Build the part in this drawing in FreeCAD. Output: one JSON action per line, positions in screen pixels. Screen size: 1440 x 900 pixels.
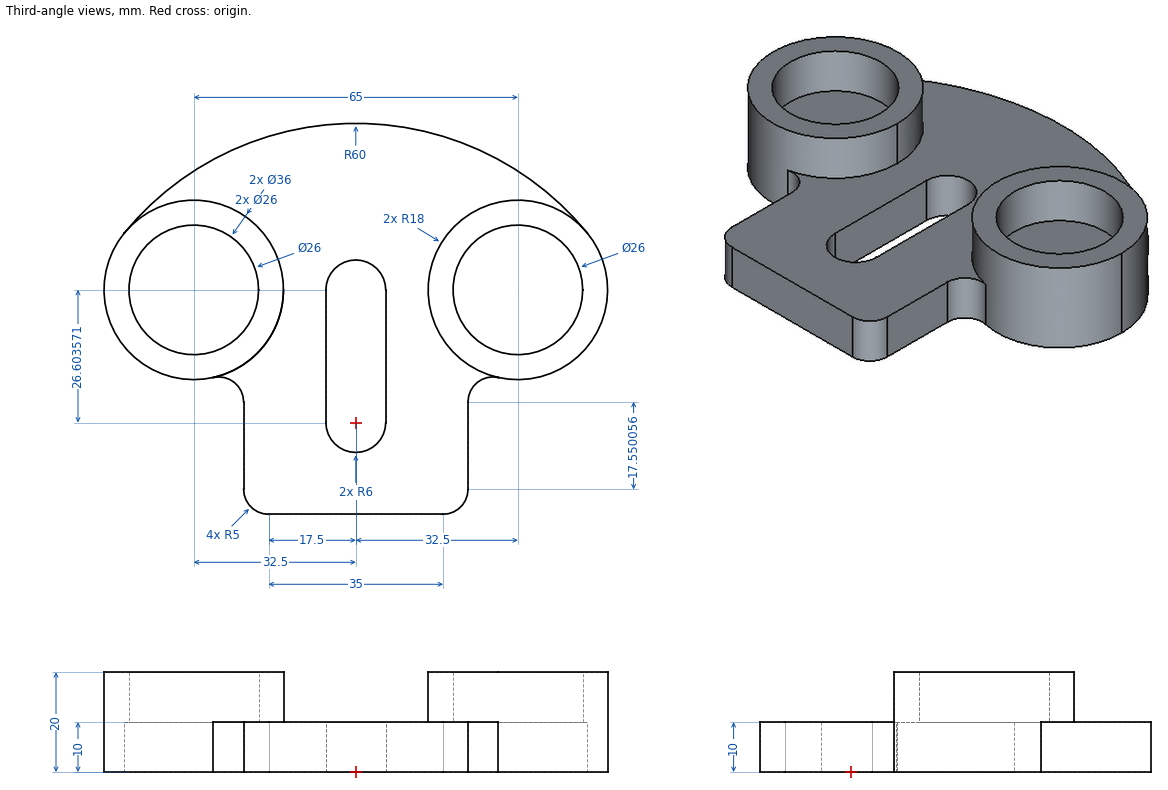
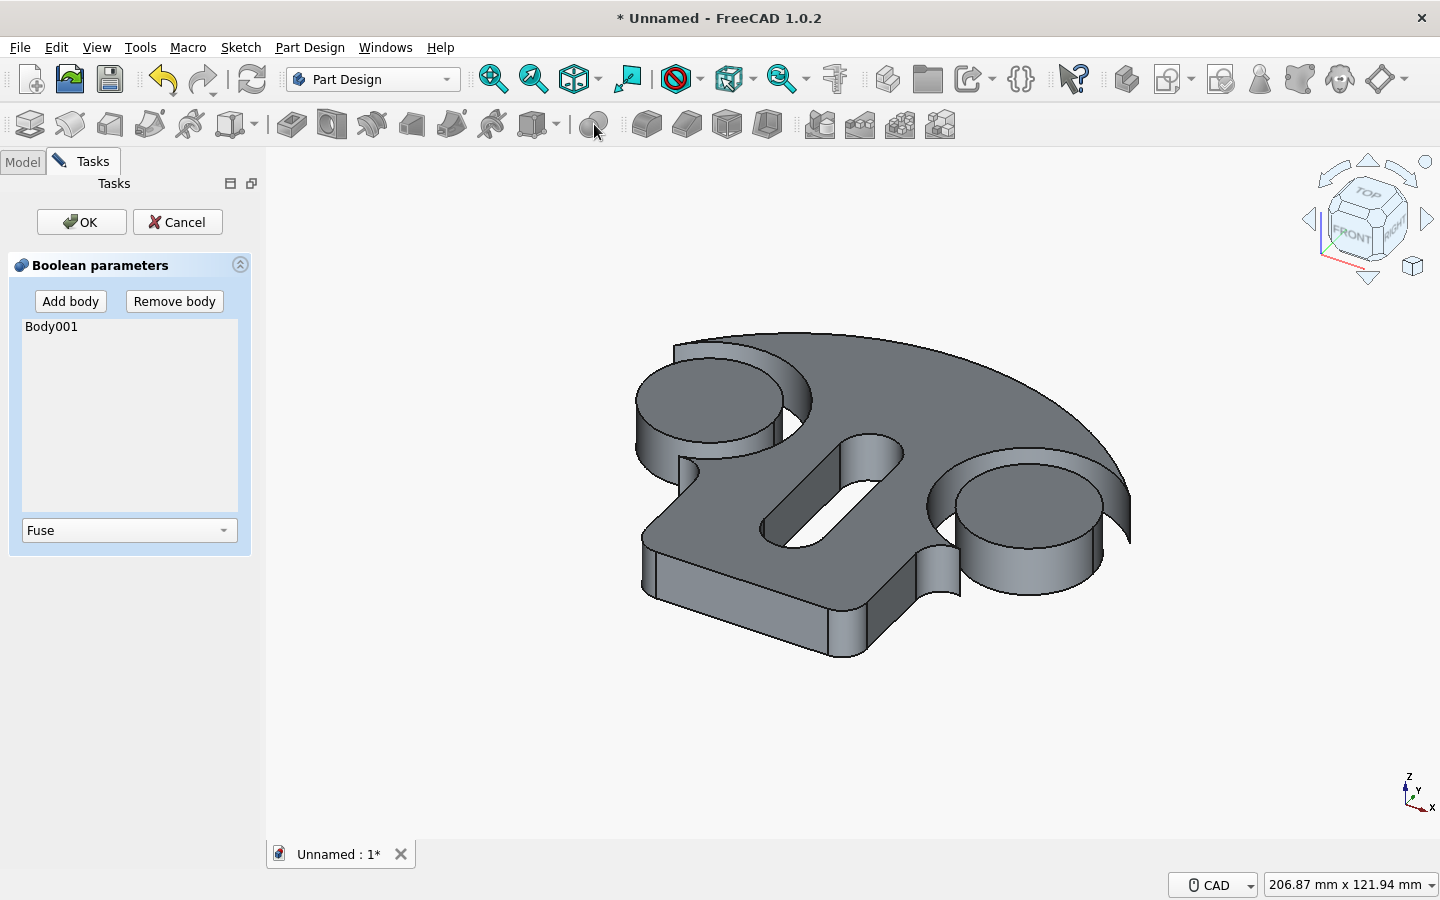
{"action": "left_click", "coordinate": [82, 222]}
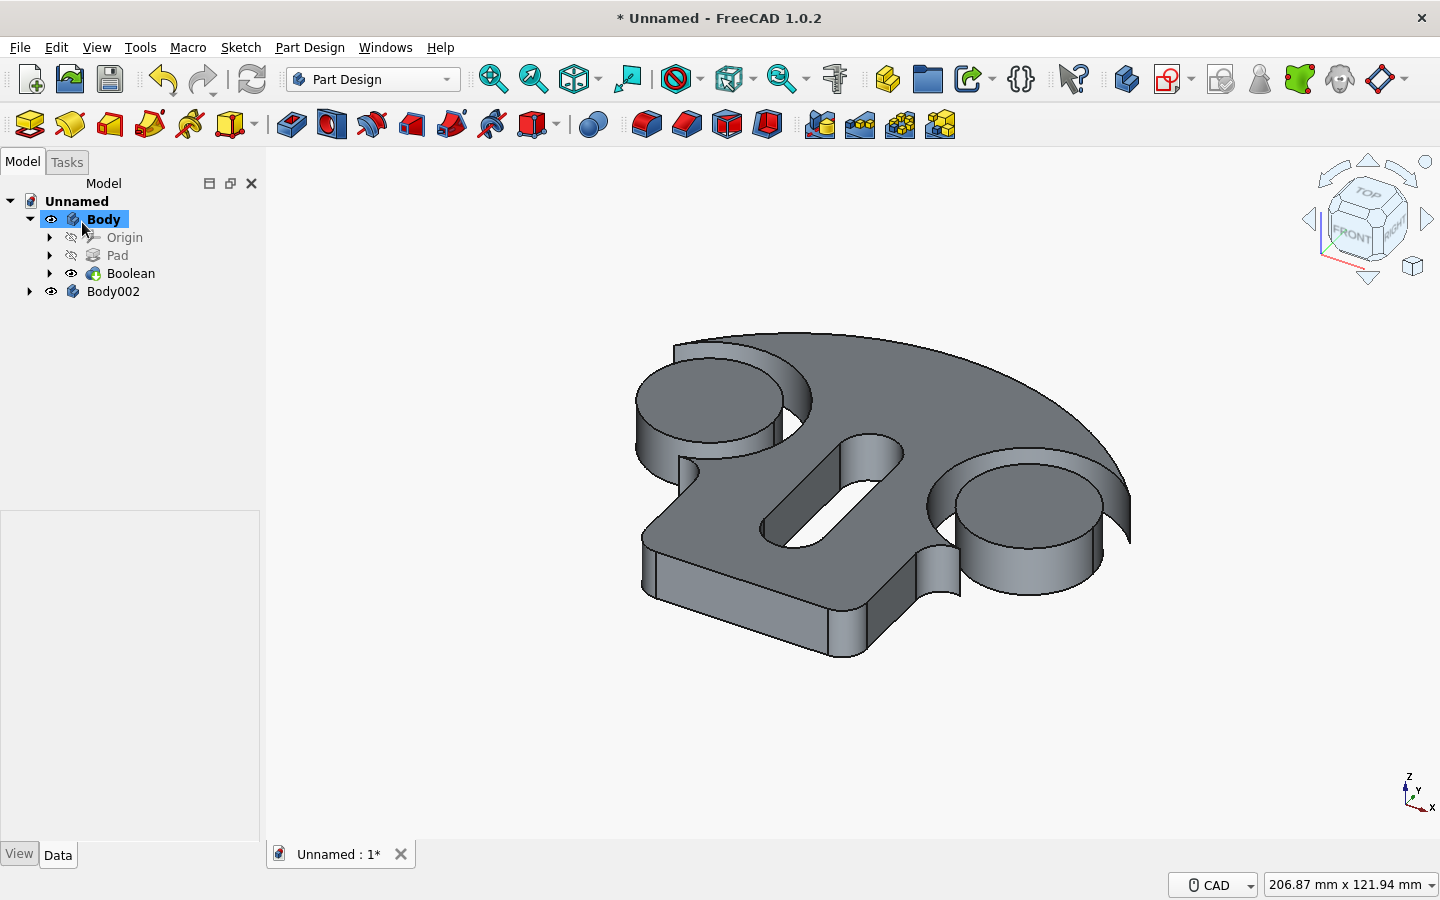
{"action": "left_click", "coordinate": [96, 291]}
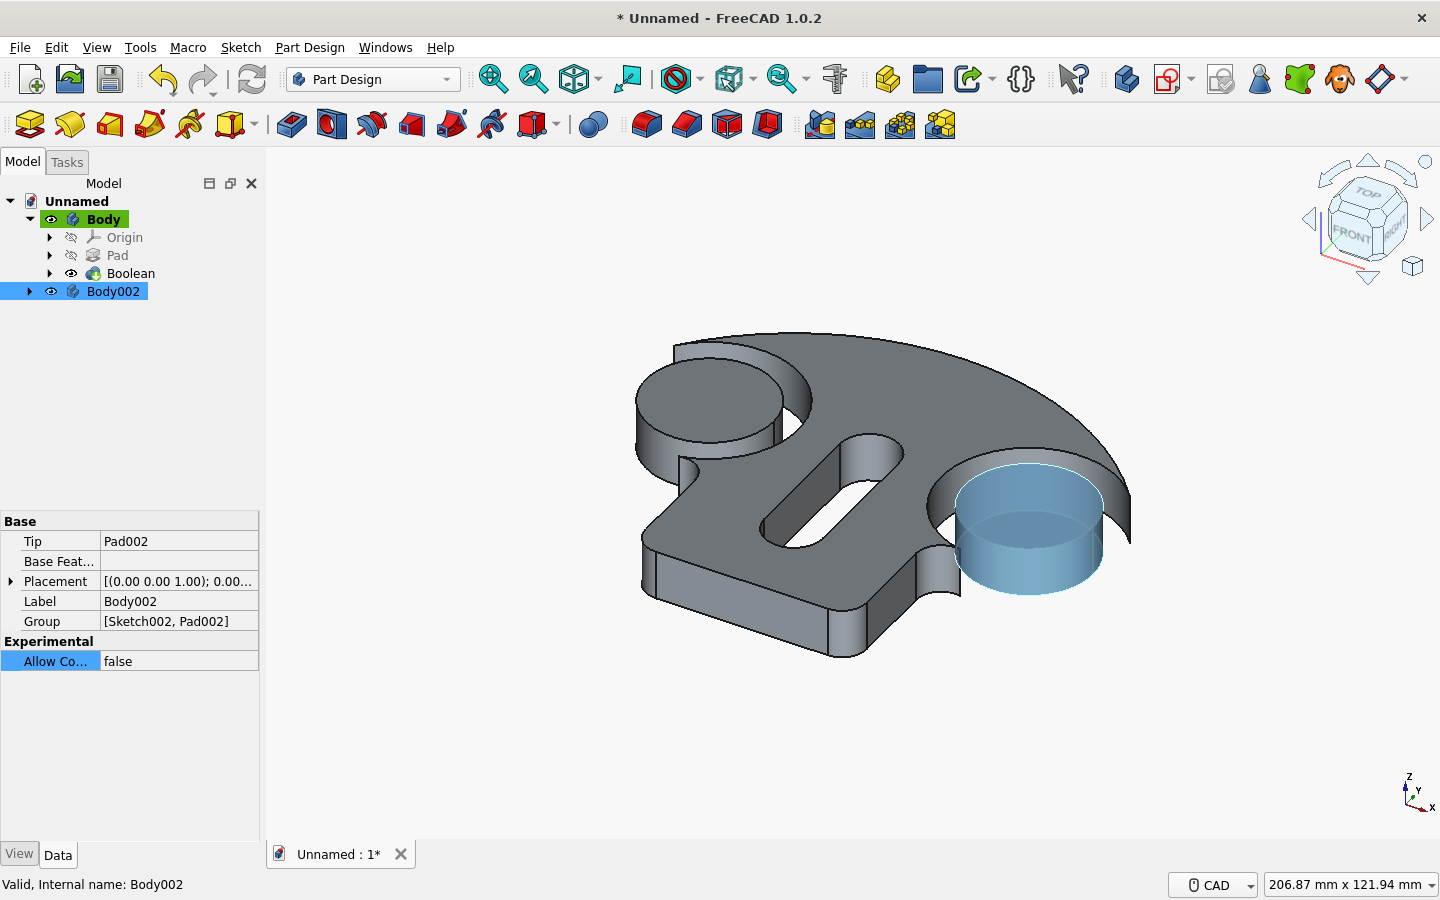
{"action": "left_click", "coordinate": [594, 124]}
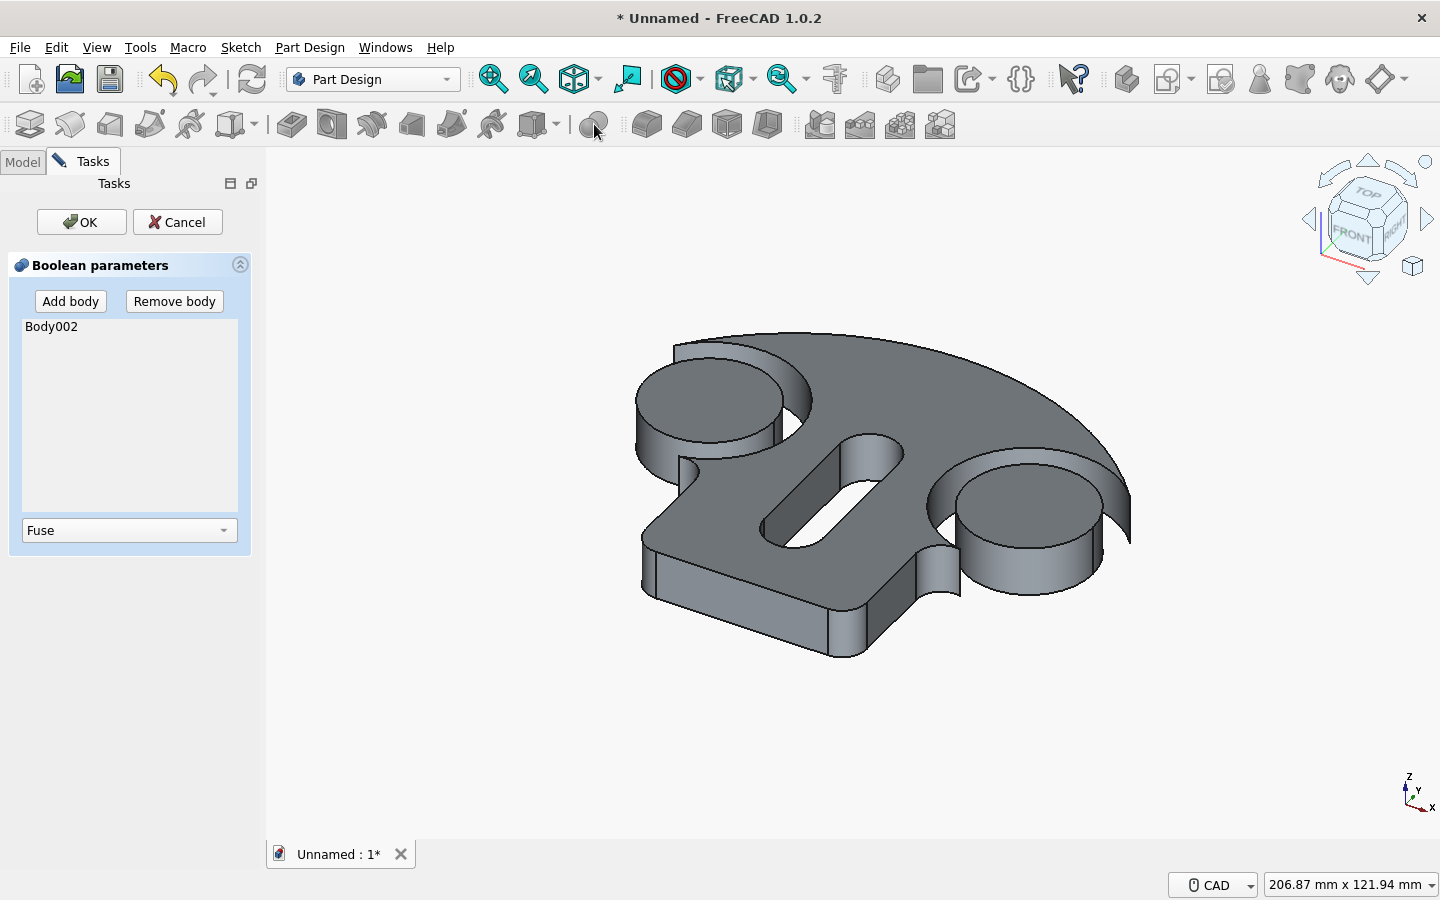
{"action": "left_click", "coordinate": [82, 222]}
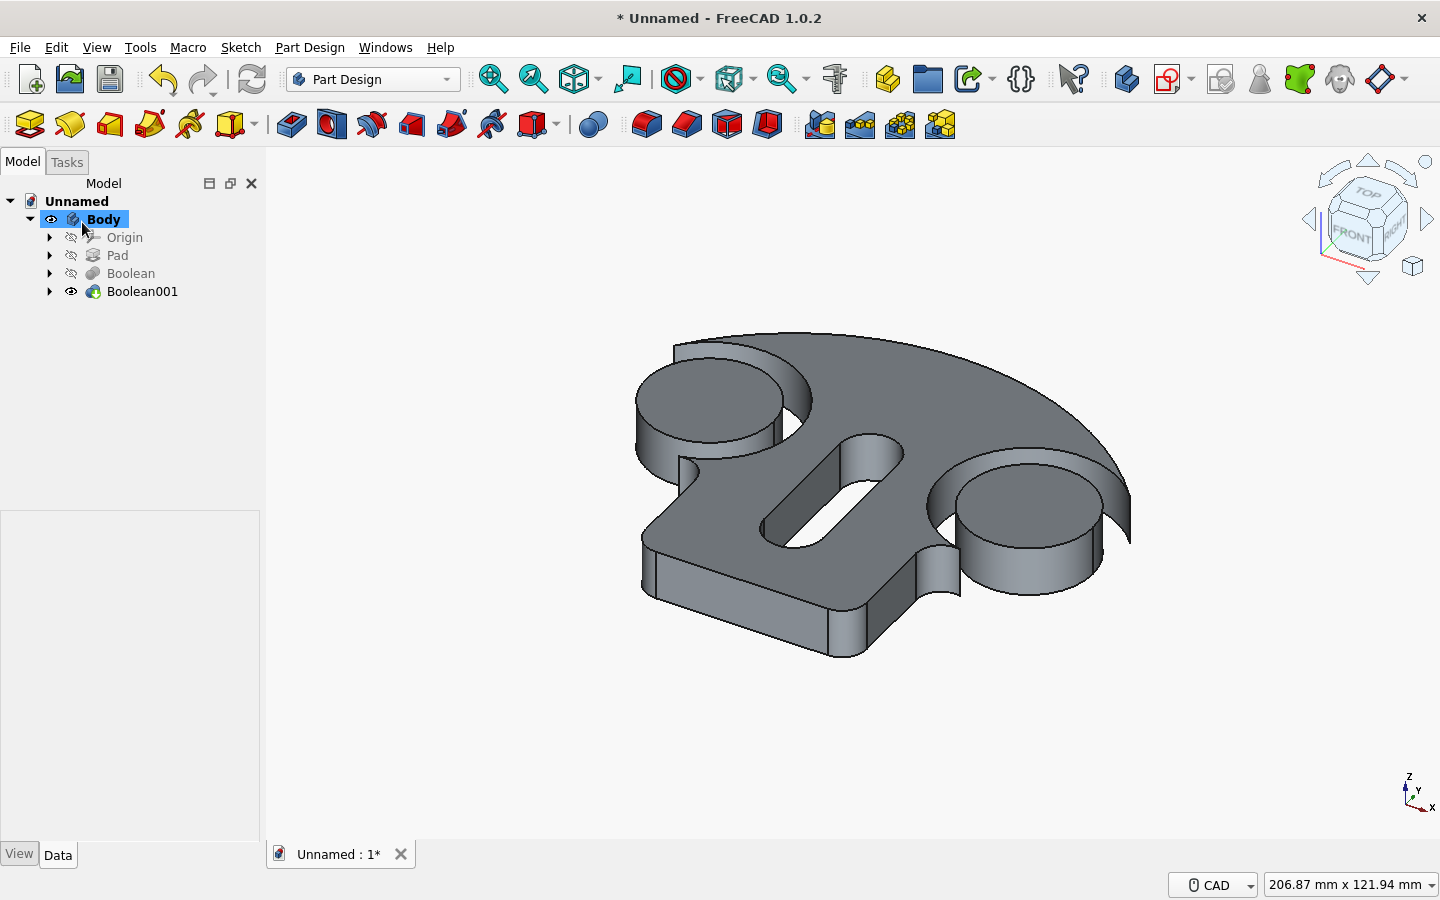
{"action": "left_click", "coordinate": [1168, 80]}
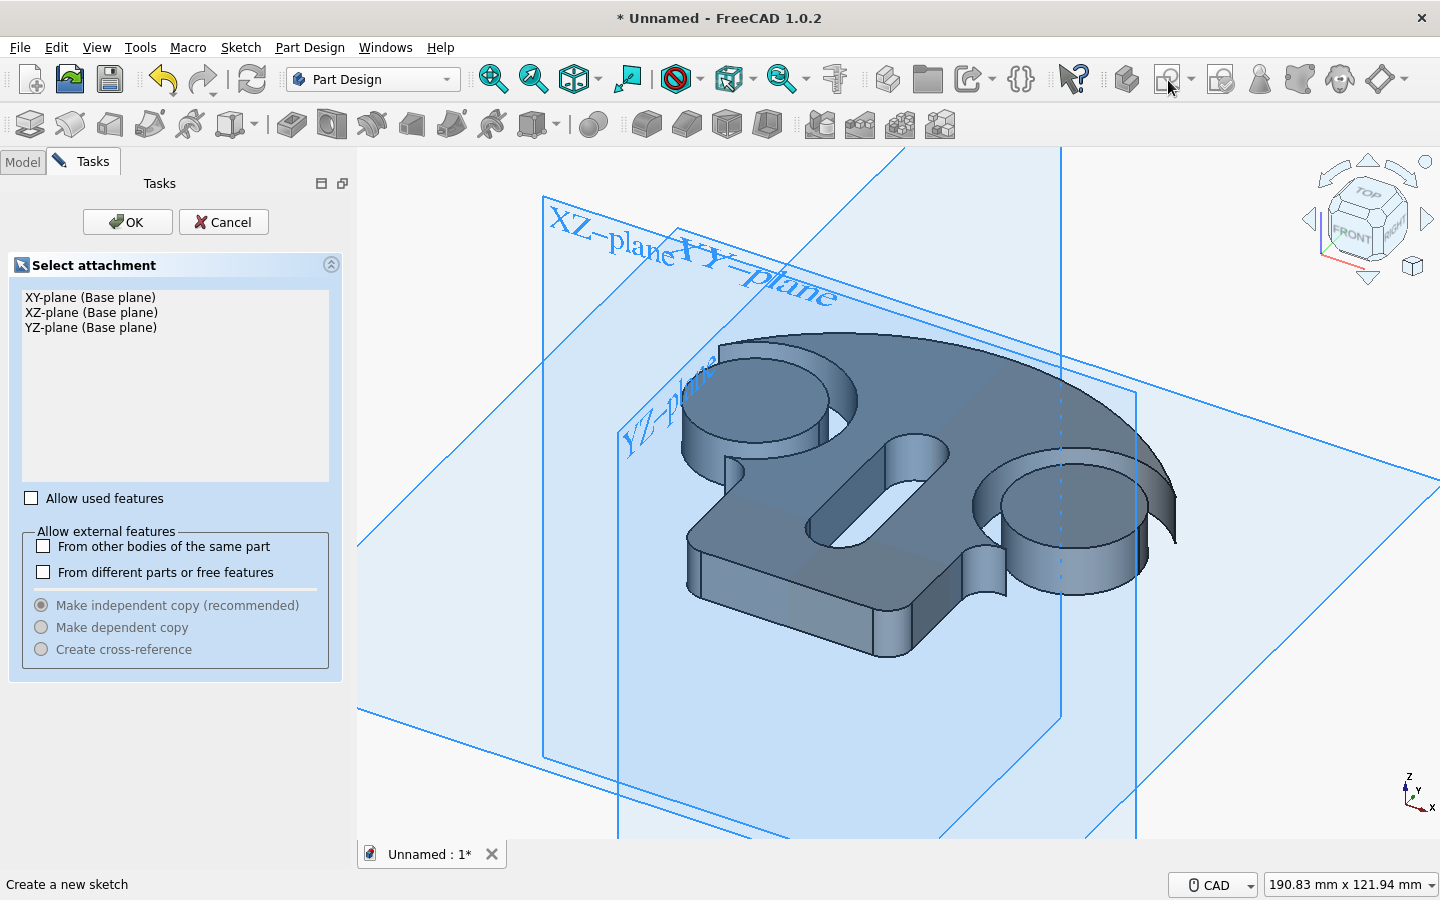
{"action": "left_click", "coordinate": [82, 298]}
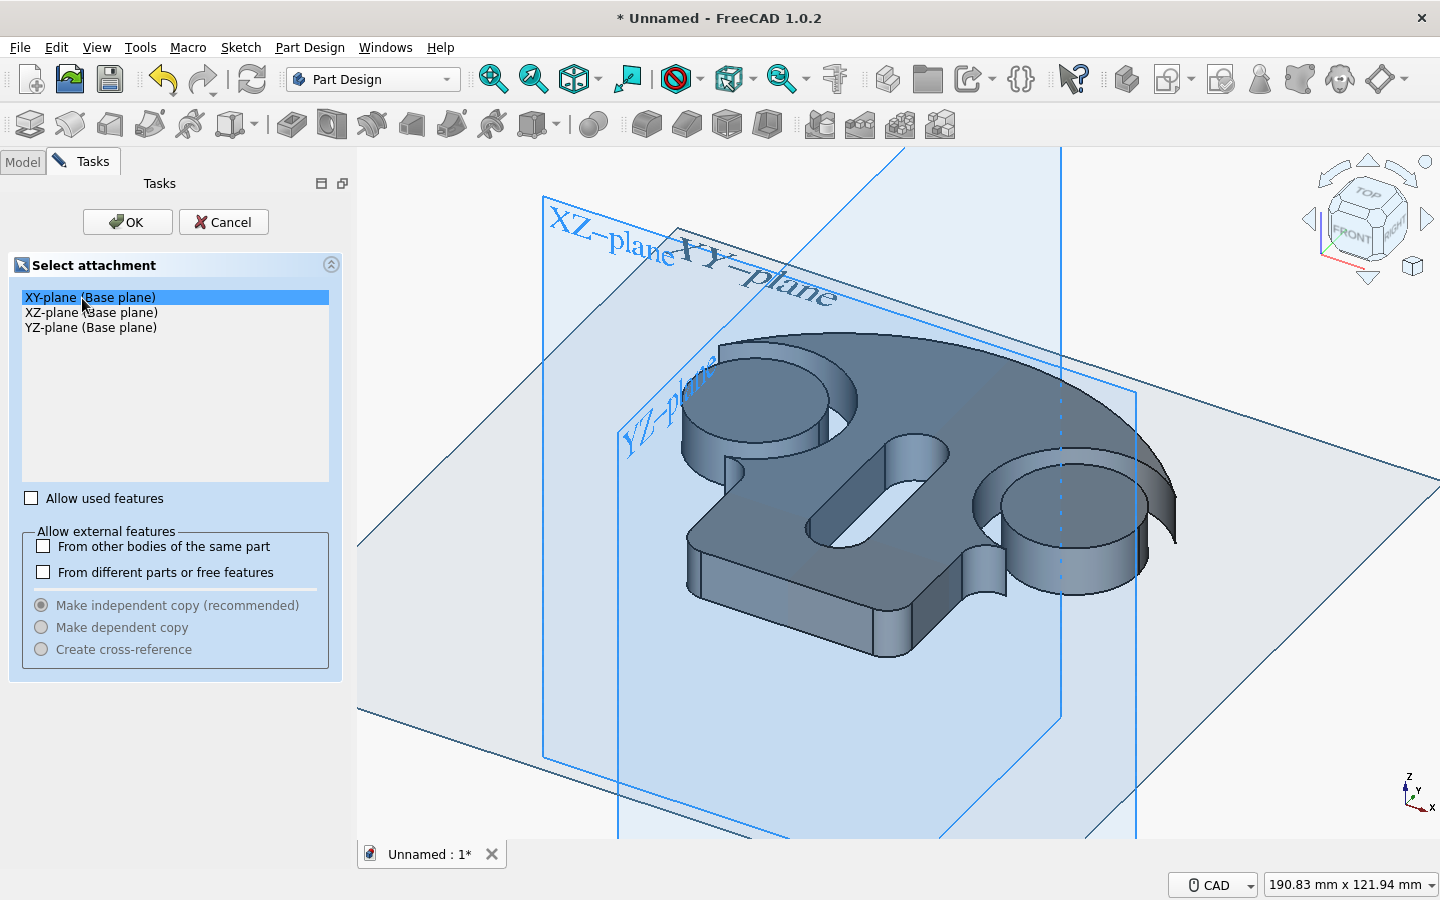
{"action": "left_click", "coordinate": [128, 222]}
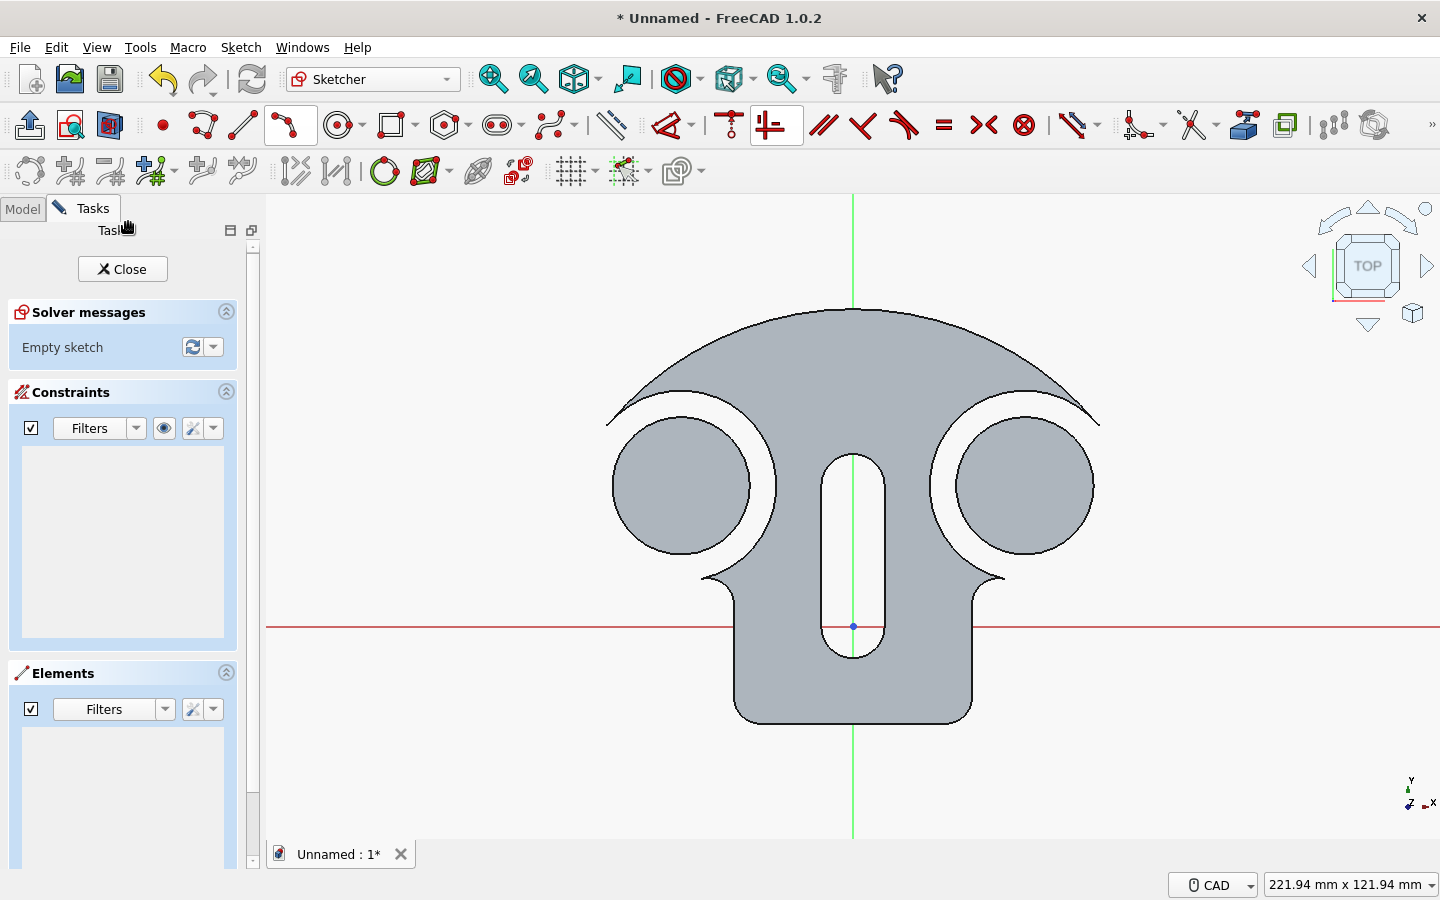
{"action": "key", "text": "q s"}